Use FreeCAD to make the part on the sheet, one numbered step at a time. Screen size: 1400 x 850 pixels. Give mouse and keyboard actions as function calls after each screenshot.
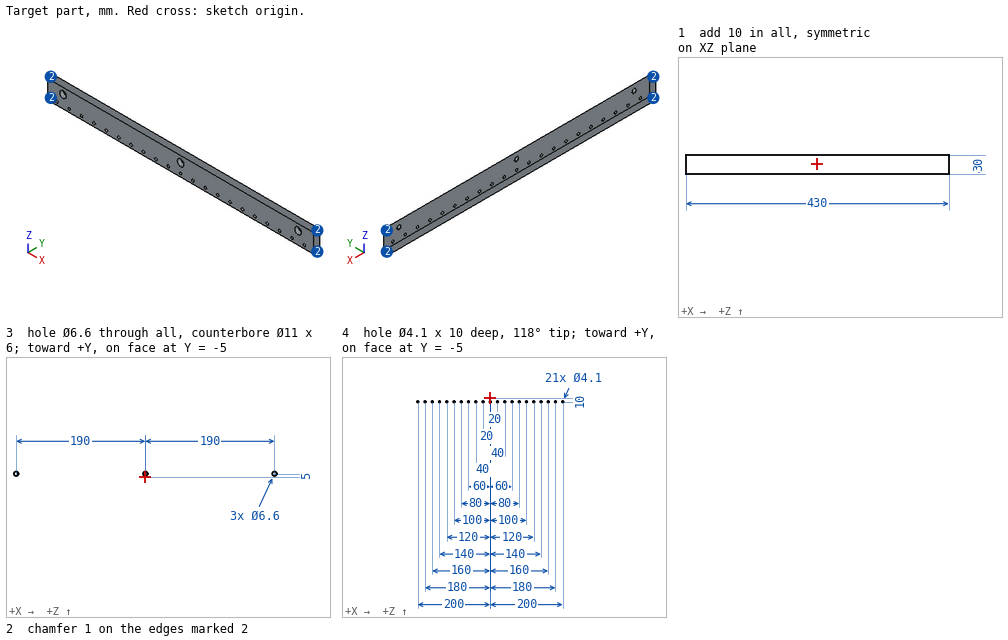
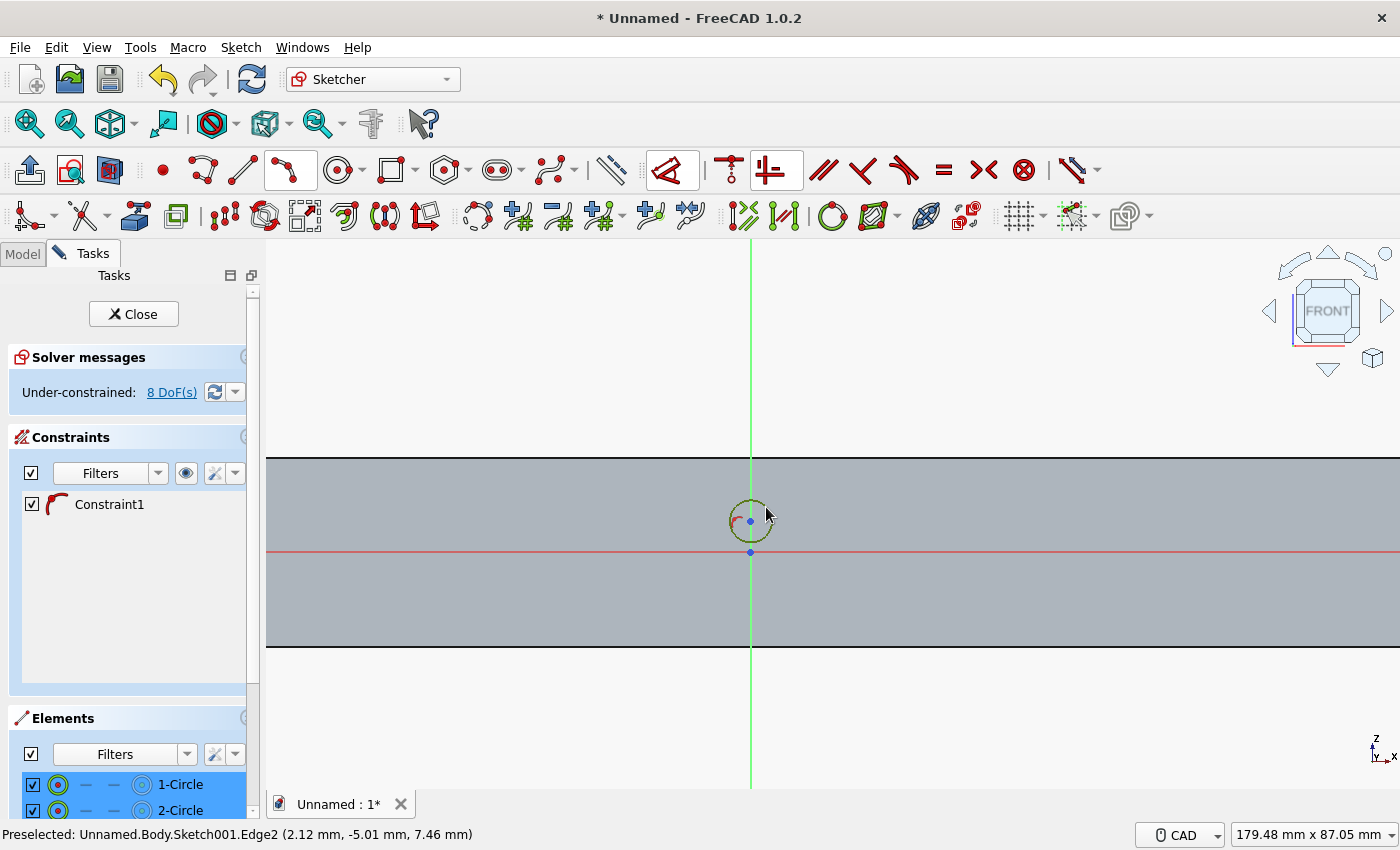
scroll(769, 510, down, 7)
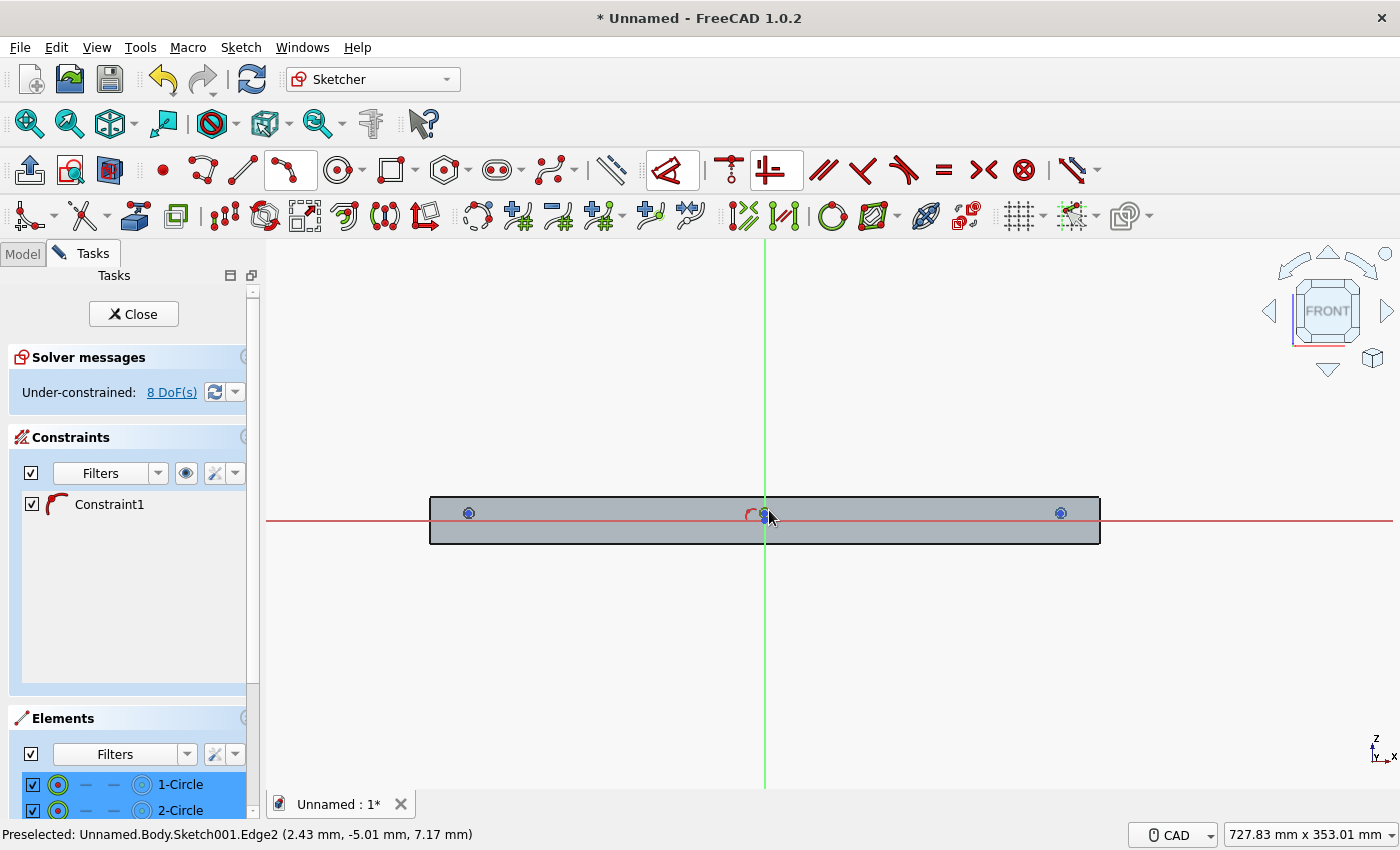
scroll(473, 510, up, 5)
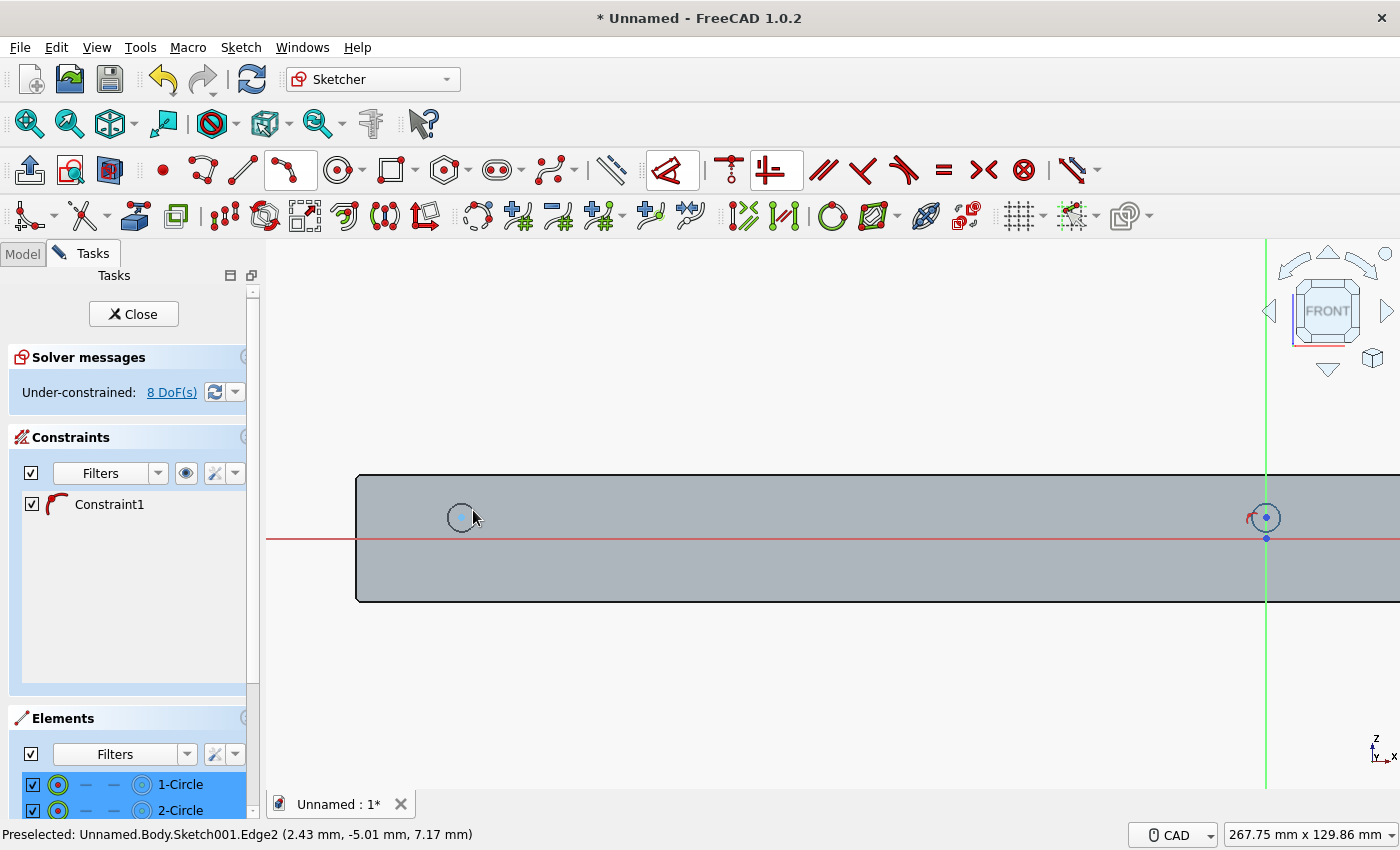
click(472, 508)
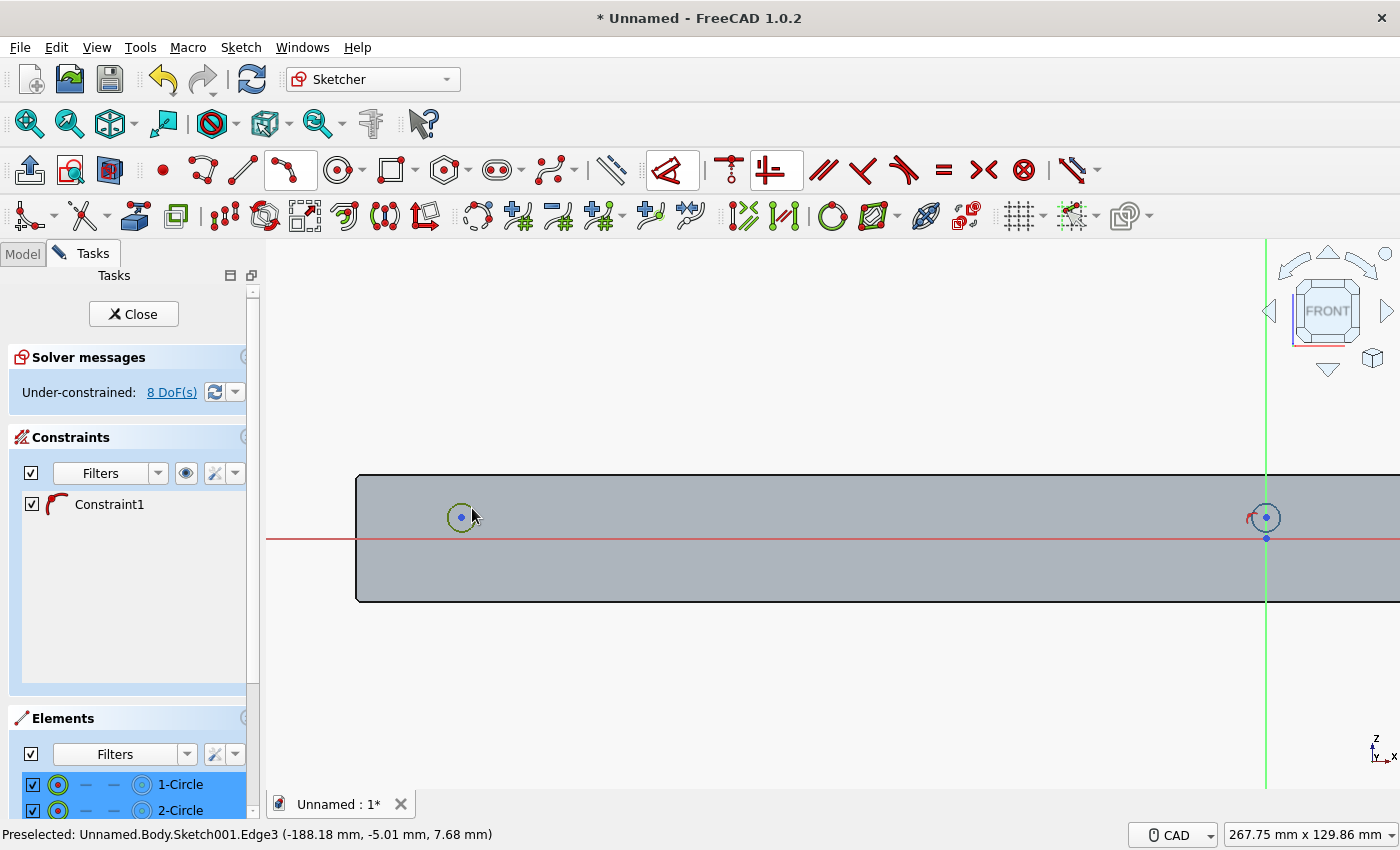
click(944, 170)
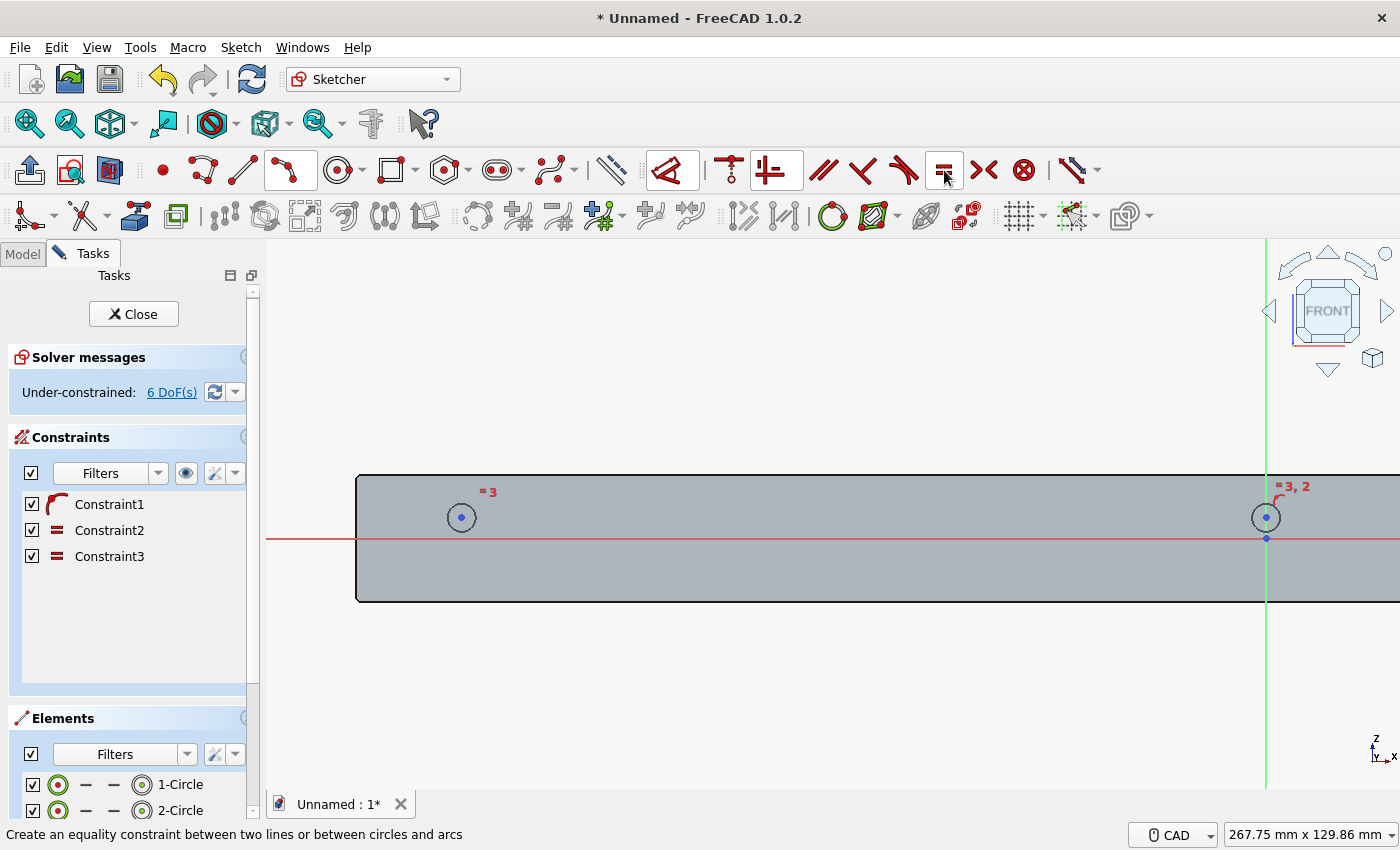
scroll(473, 510, down, 5)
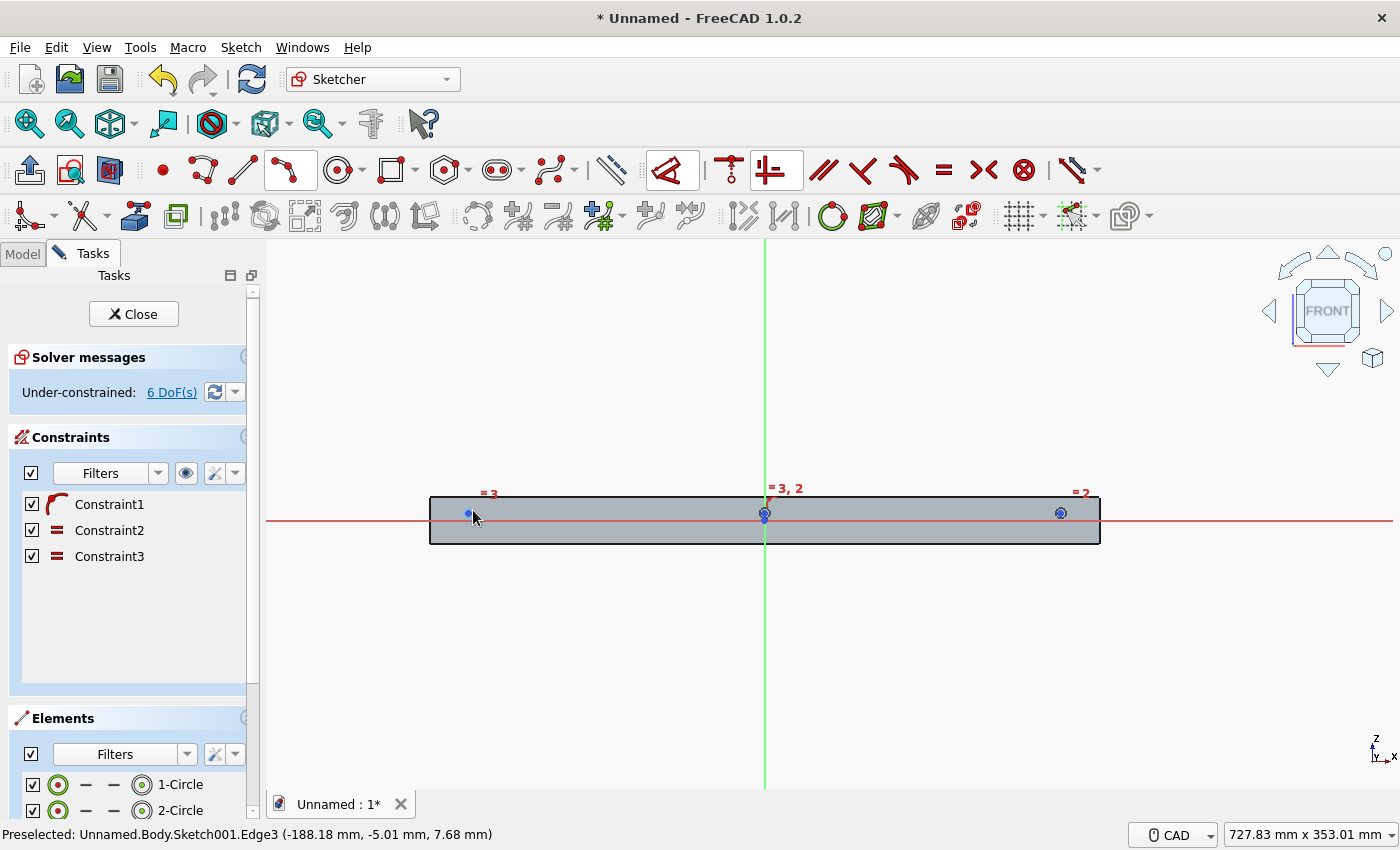
click(1061, 513)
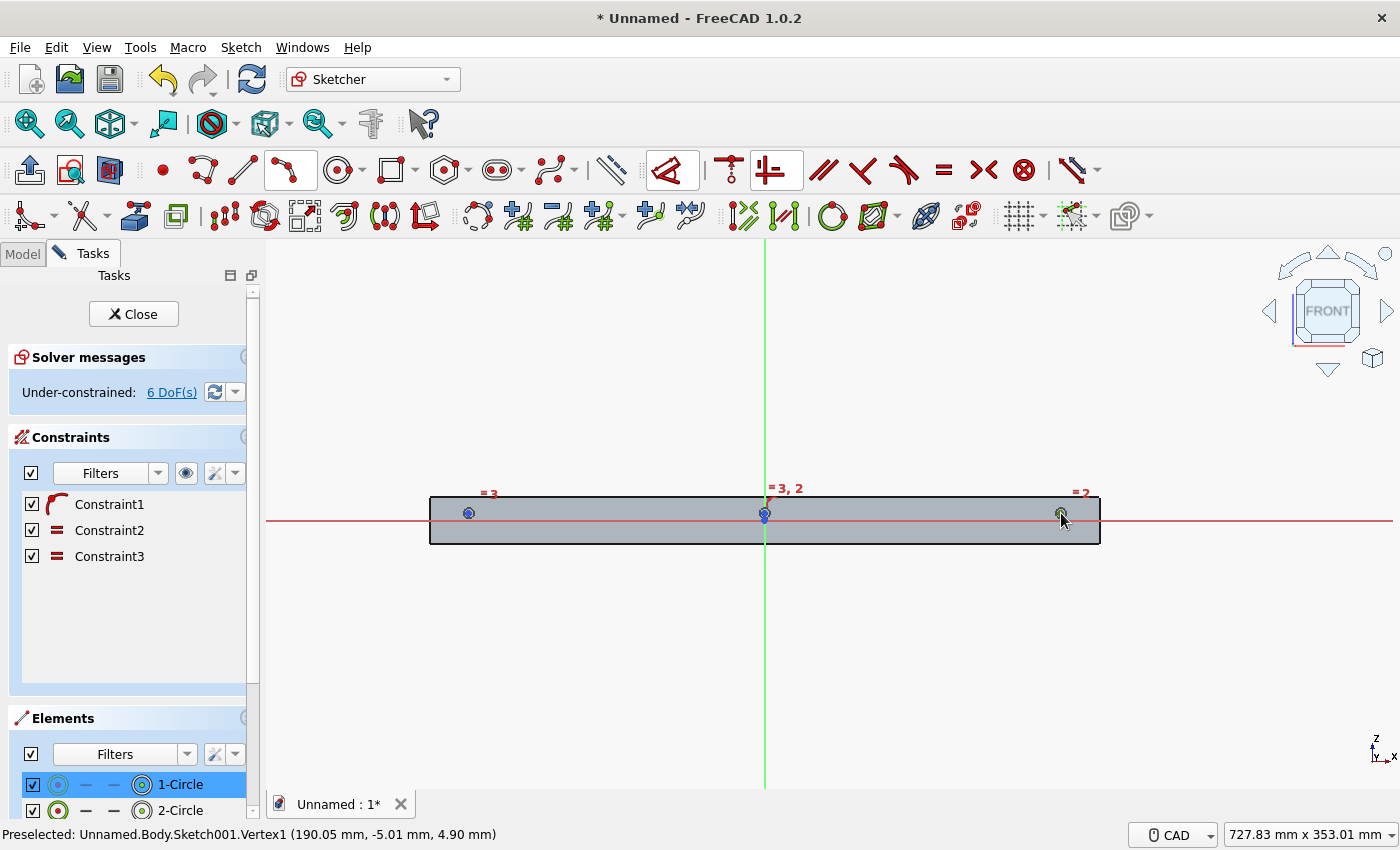
scroll(765, 513, up, 3)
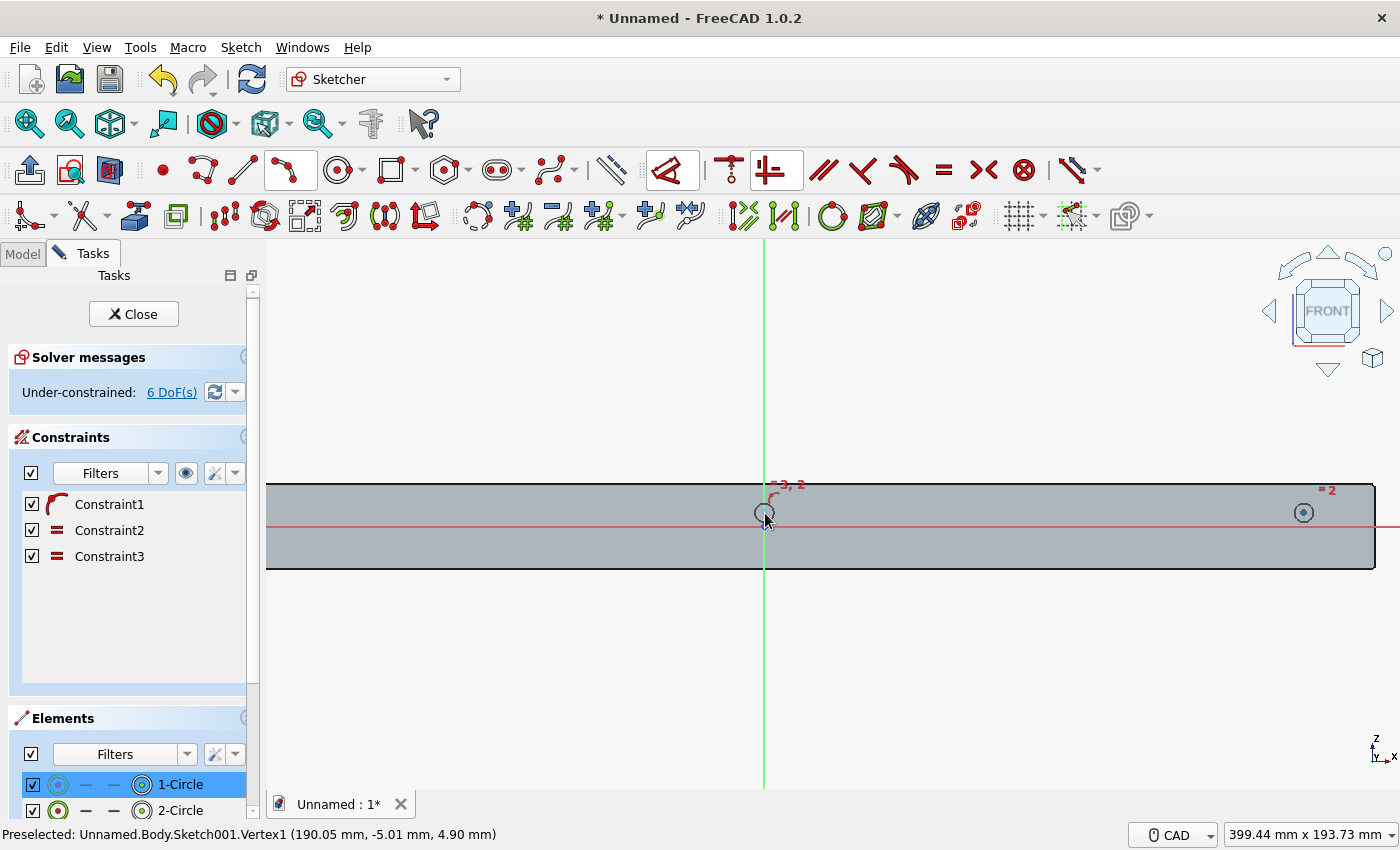
click(764, 513)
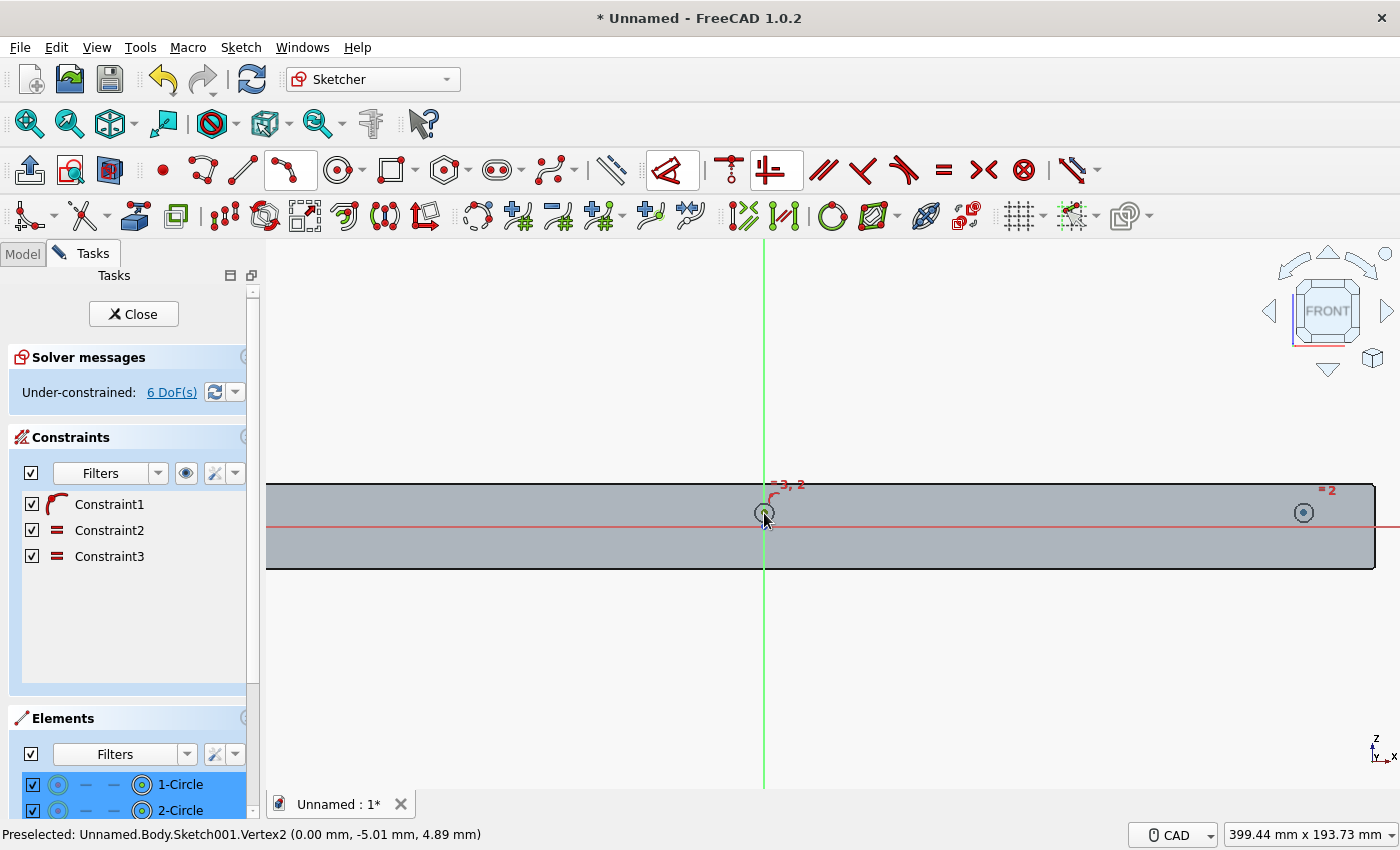
key(h)